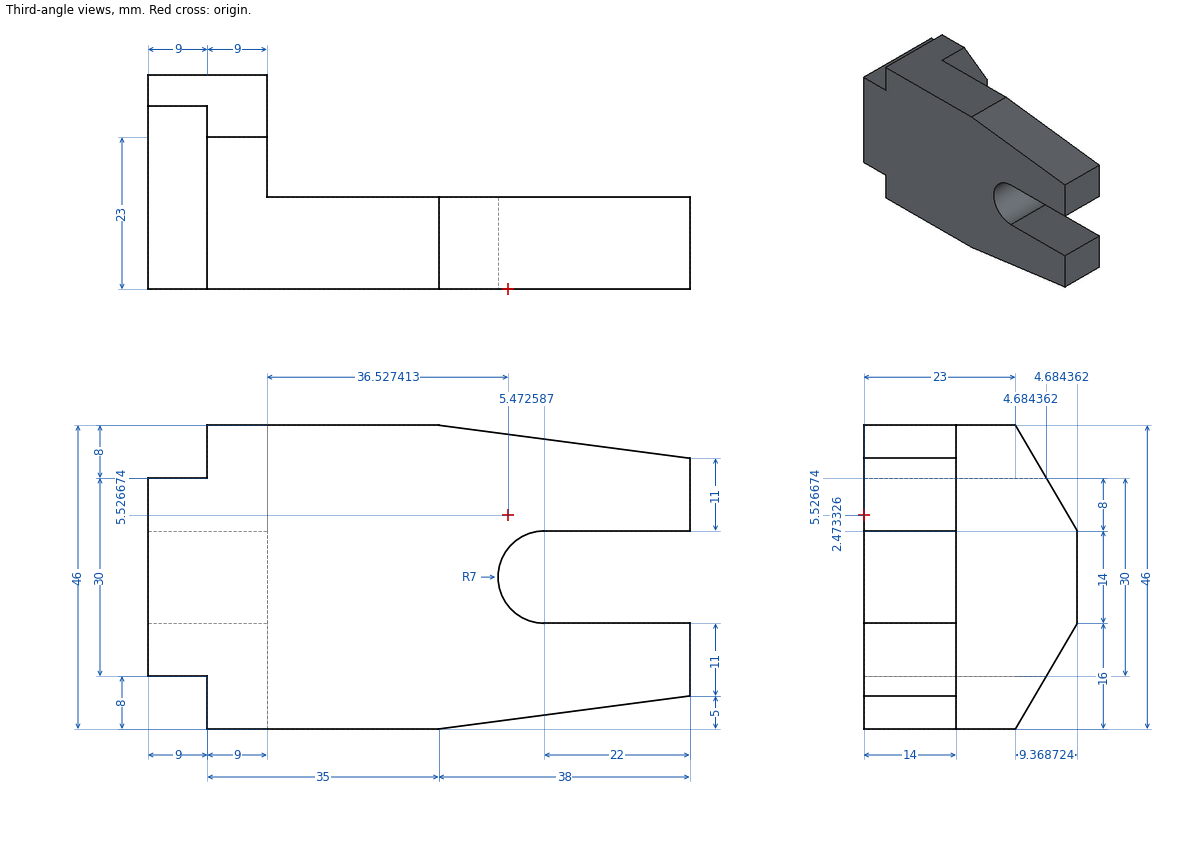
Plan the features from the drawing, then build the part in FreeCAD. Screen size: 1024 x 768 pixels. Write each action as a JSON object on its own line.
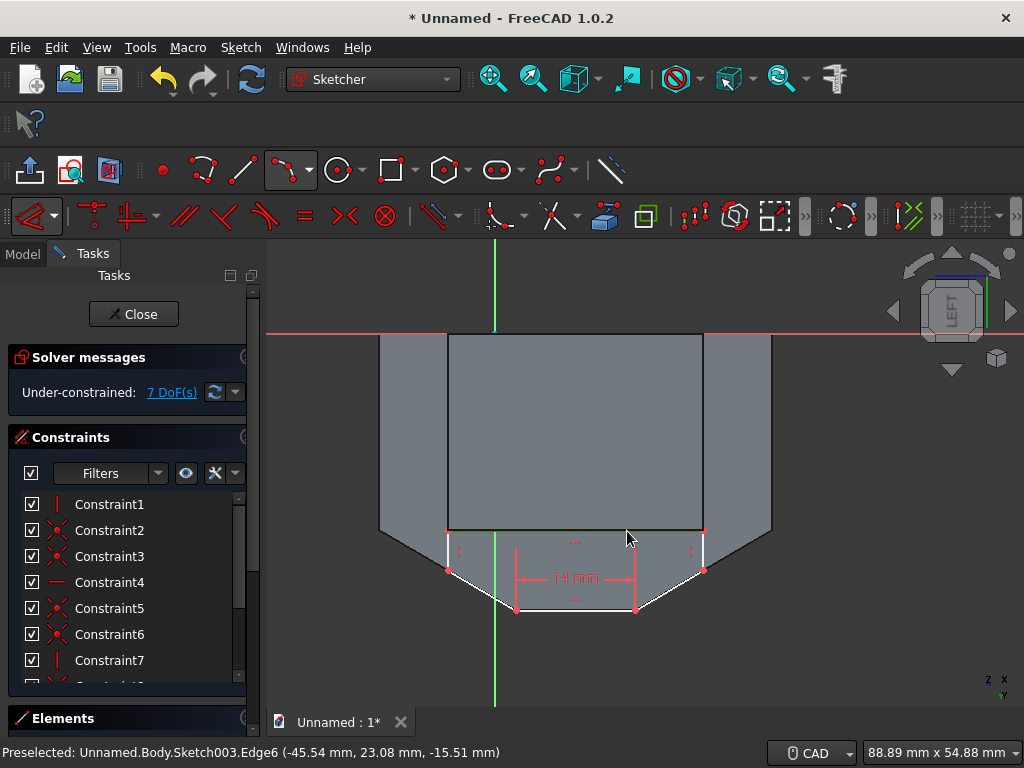
{"action": "key", "text": "l"}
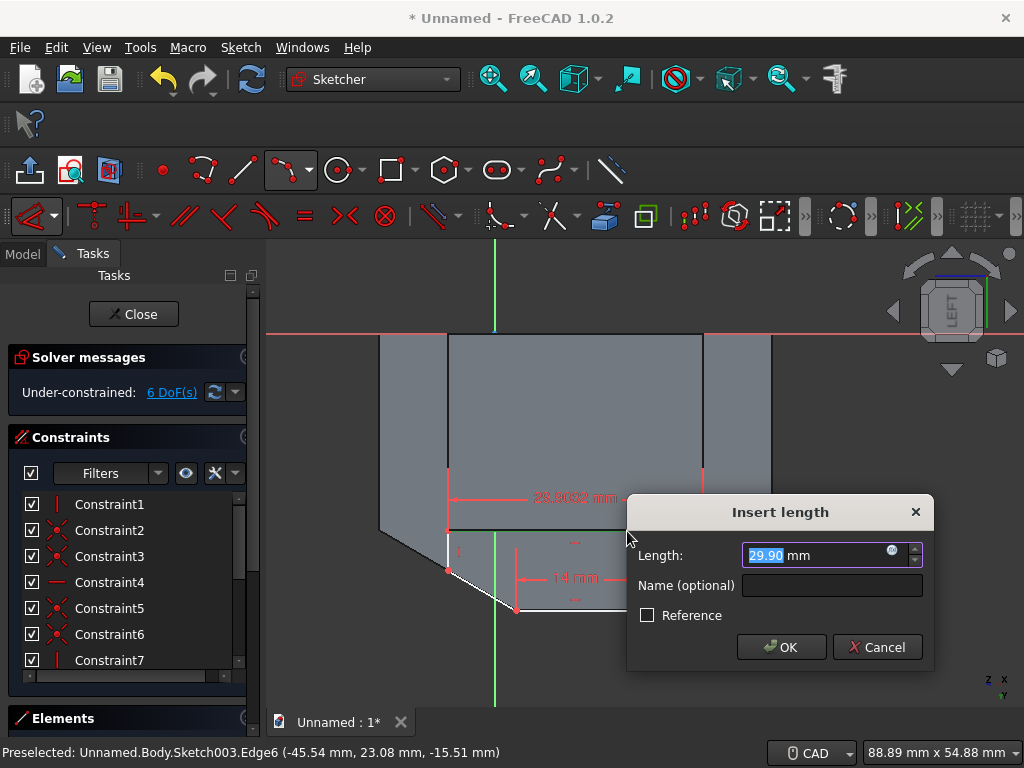
{"action": "type", "text": "30"}
{"action": "key", "text": "Return"}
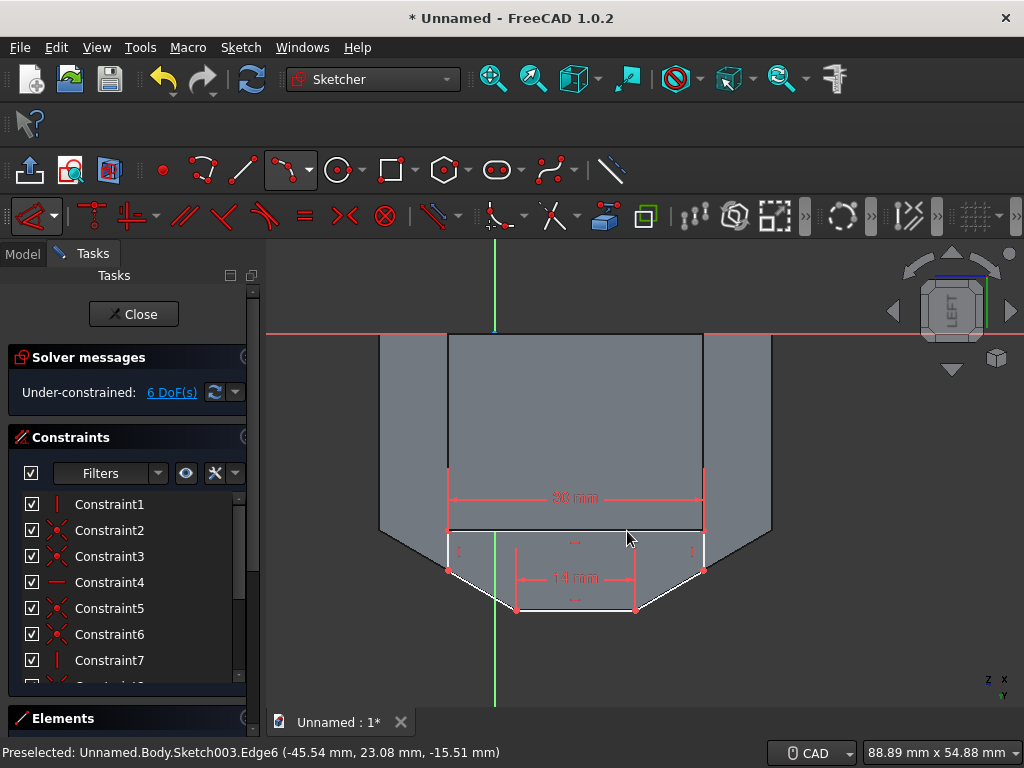
{"action": "left_click", "coordinate": [468, 583]}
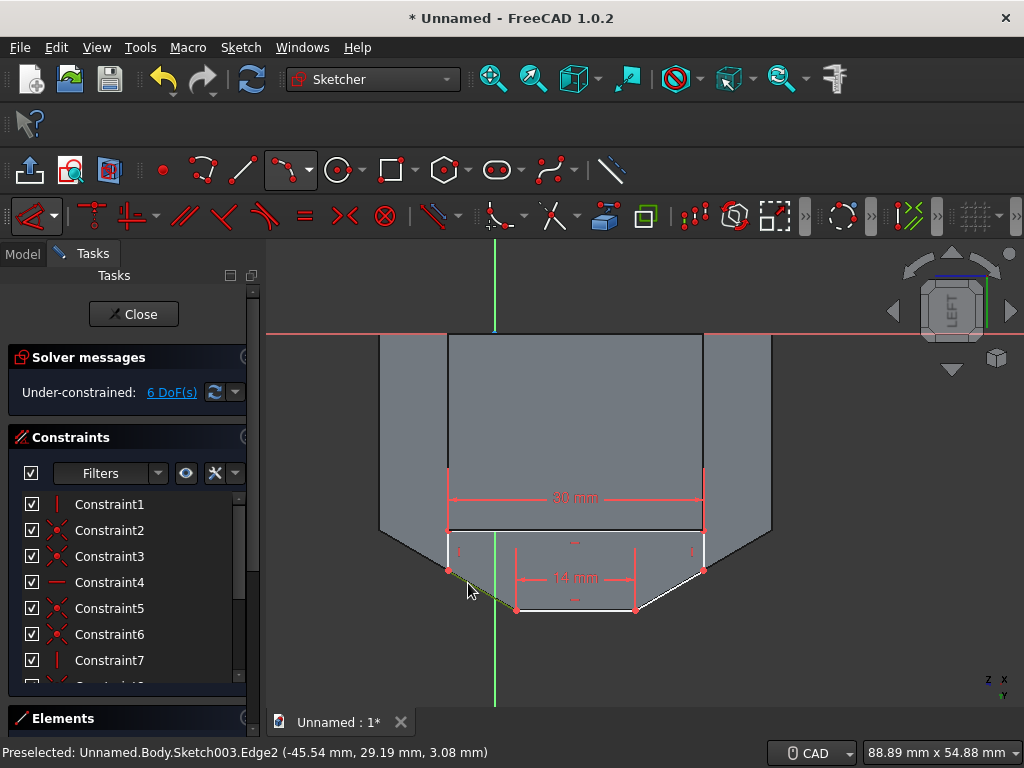
{"action": "left_click", "coordinate": [56, 216]}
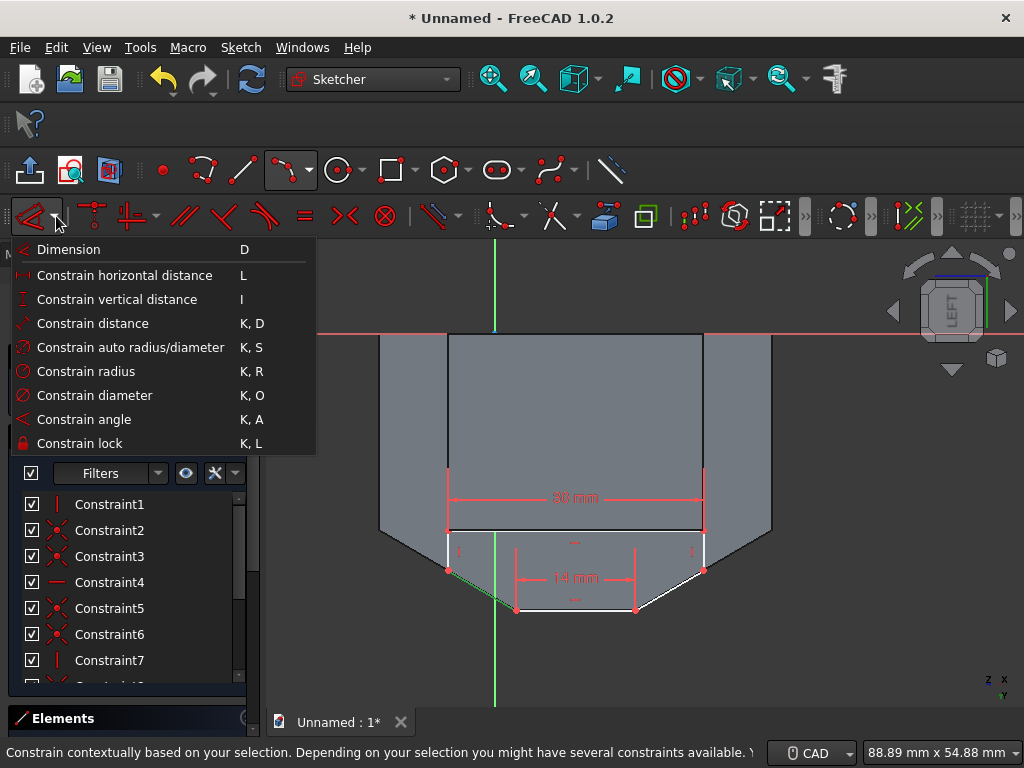
{"action": "left_click", "coordinate": [164, 275]}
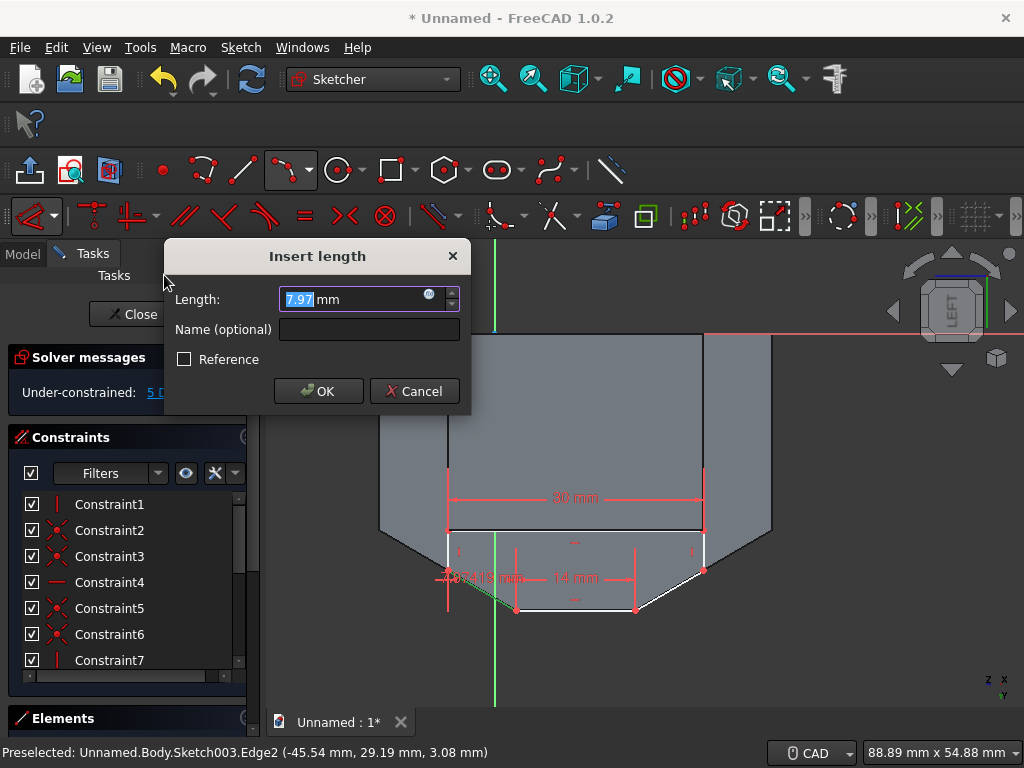
{"action": "type", "text": "8"}
{"action": "key", "text": "Return"}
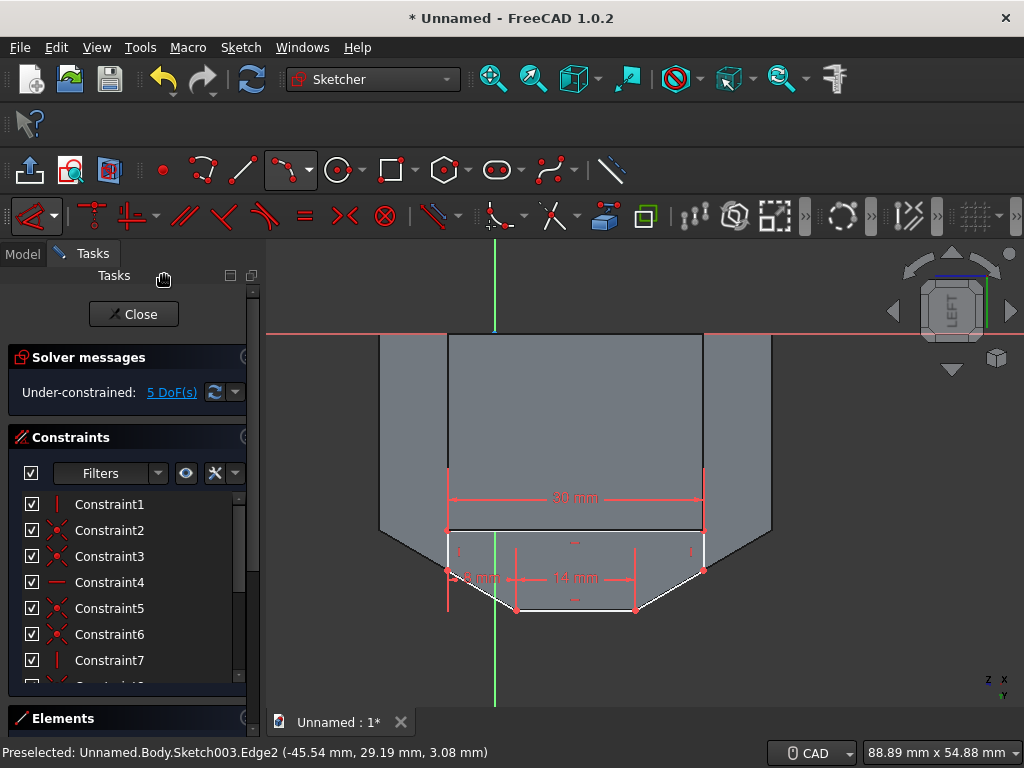
{"action": "left_click", "coordinate": [448, 531]}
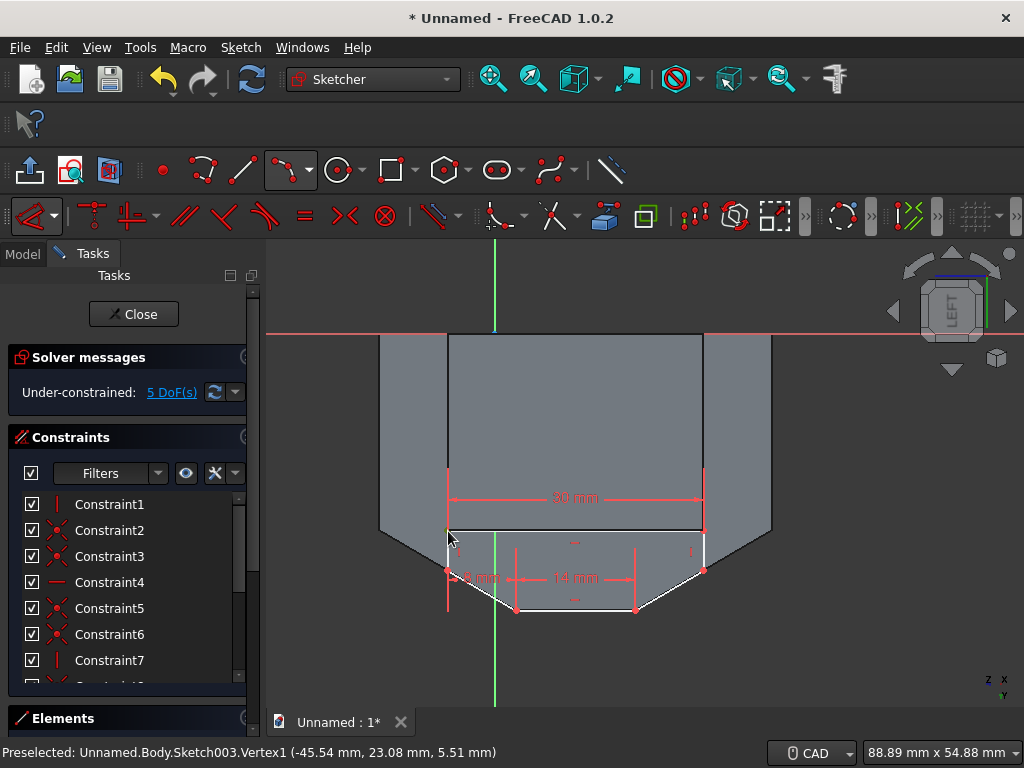
{"action": "left_click", "coordinate": [56, 216]}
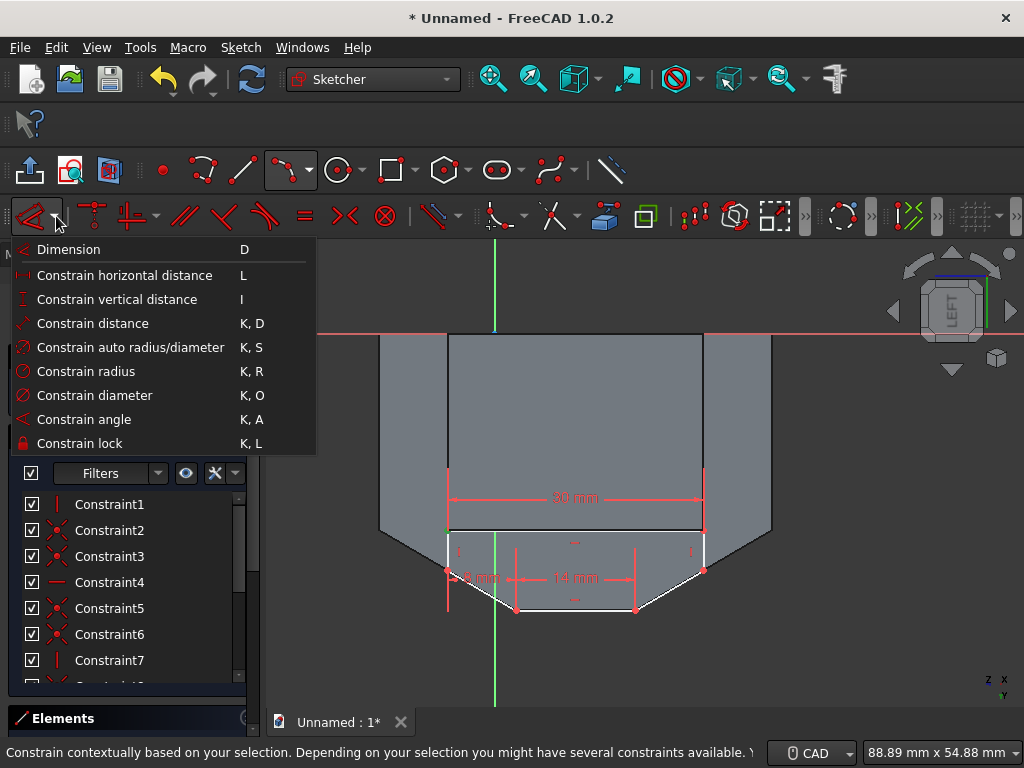
{"action": "left_click", "coordinate": [164, 299]}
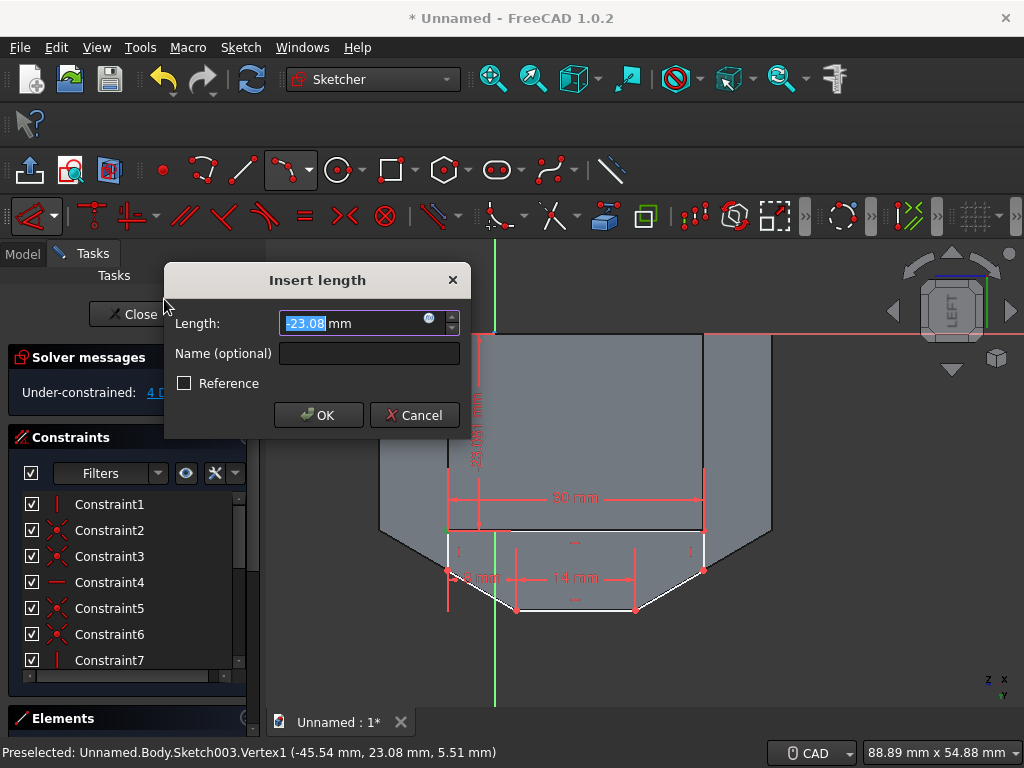
{"action": "type", "text": "-23"}
{"action": "key", "text": "Return"}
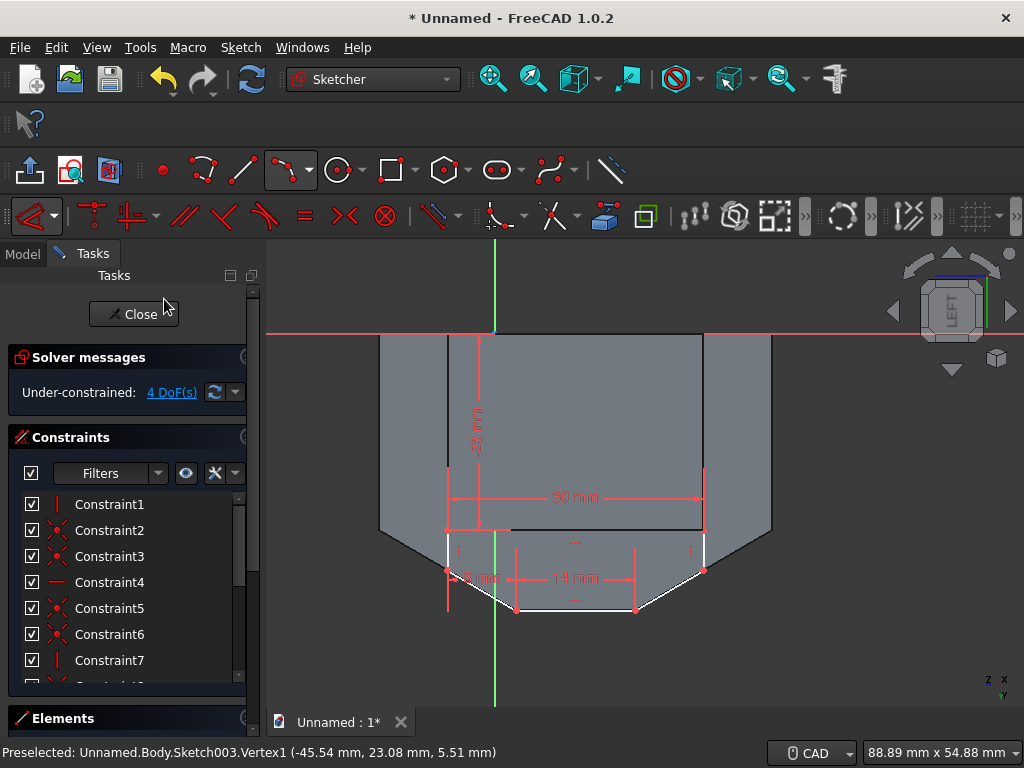
{"action": "left_click", "coordinate": [448, 543]}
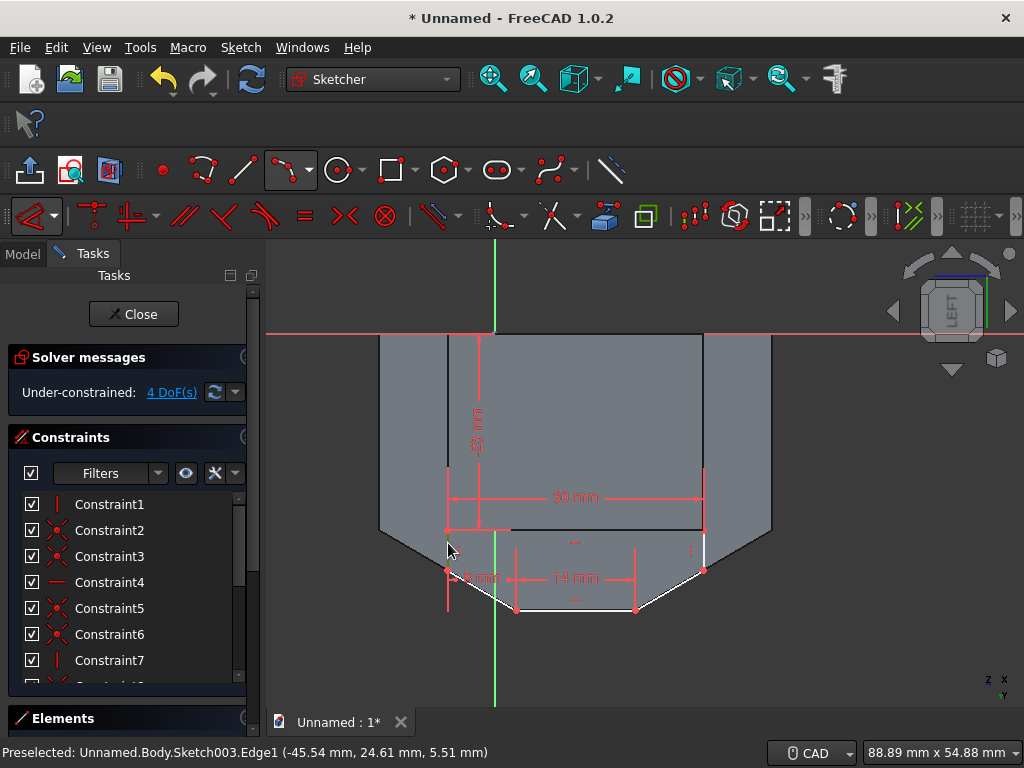
{"action": "left_click", "coordinate": [56, 216]}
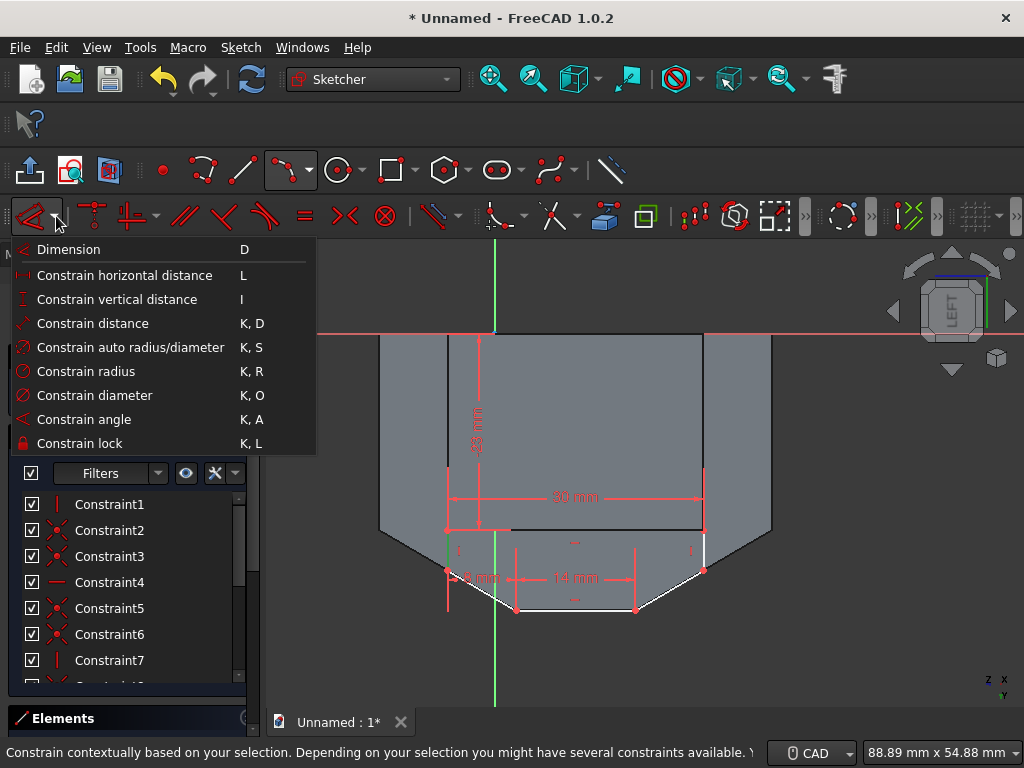
{"action": "left_click", "coordinate": [164, 299]}